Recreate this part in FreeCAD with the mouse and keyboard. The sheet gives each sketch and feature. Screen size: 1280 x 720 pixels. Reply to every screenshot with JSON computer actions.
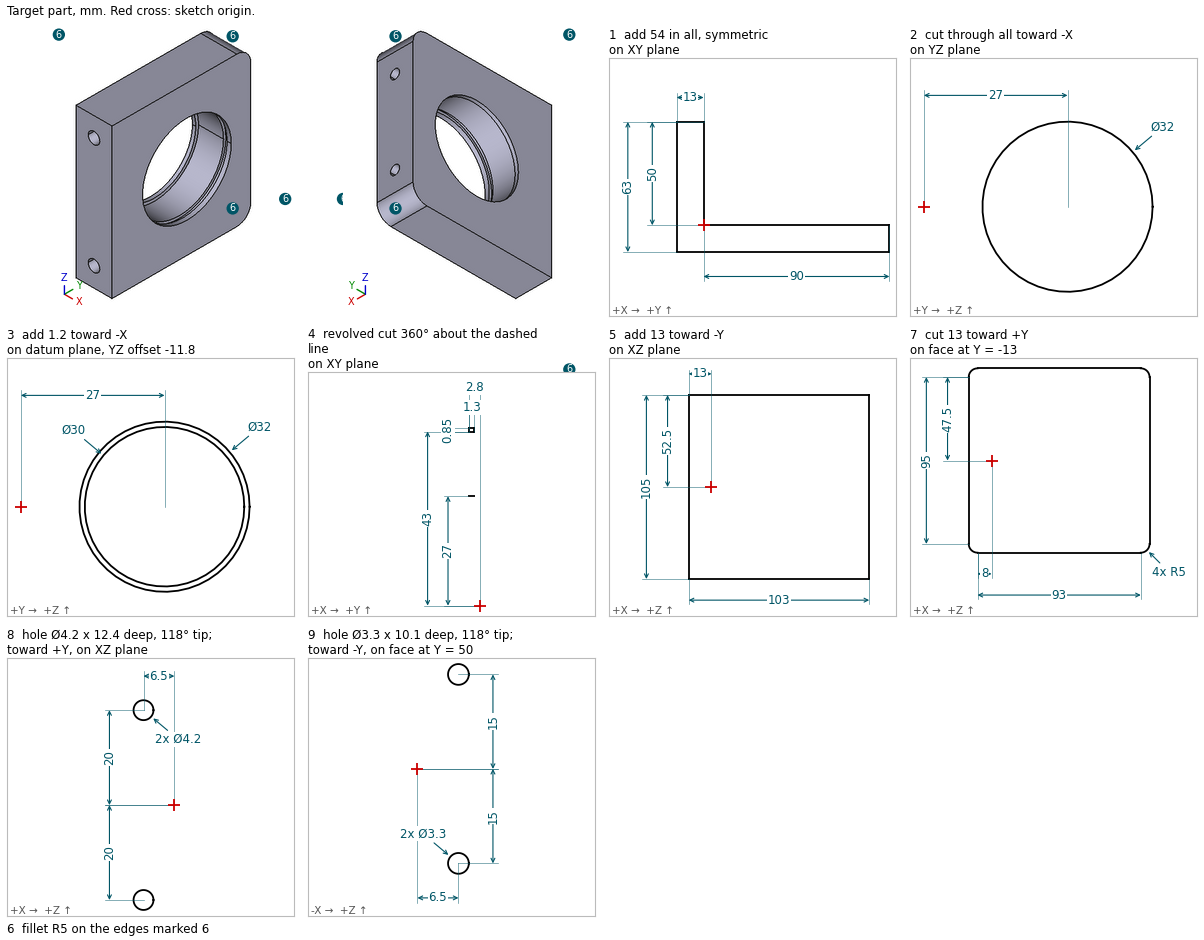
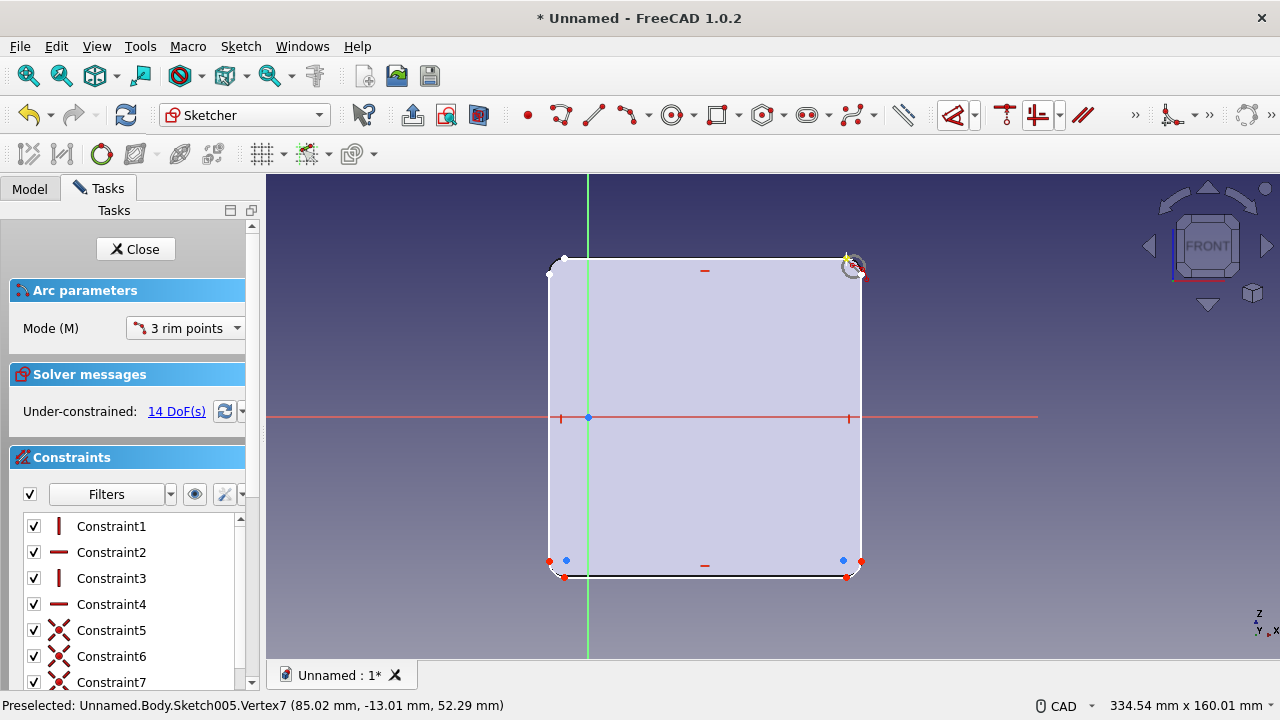
{"action": "scroll", "coordinate": [857, 263], "scroll_direction": "up", "scroll_amount": 7}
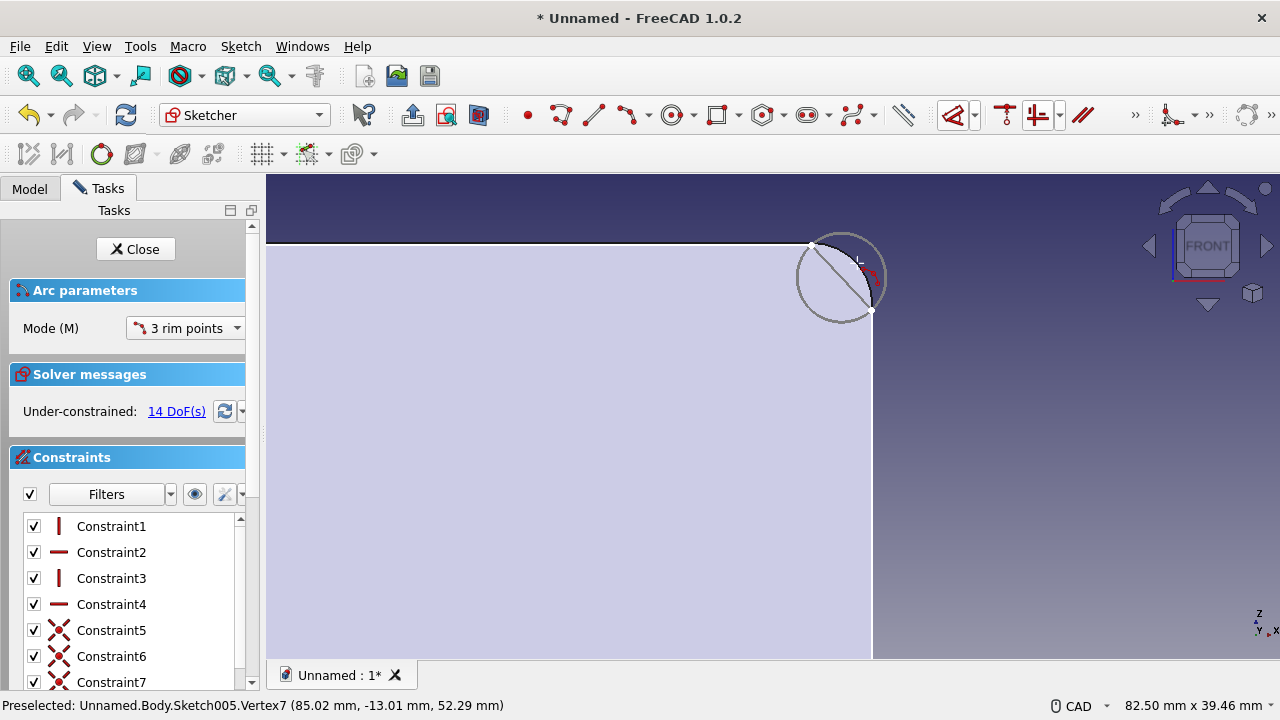
{"action": "left_click", "coordinate": [854, 261]}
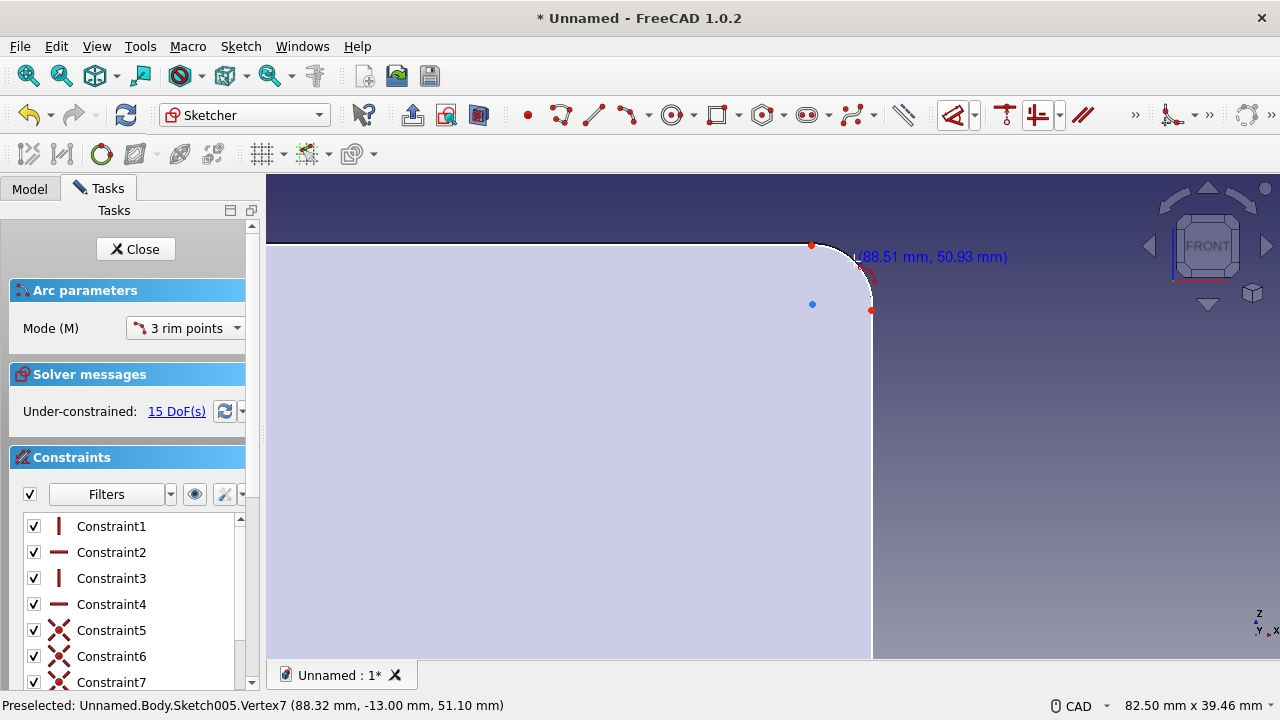
{"action": "scroll", "coordinate": [857, 262], "scroll_direction": "down", "scroll_amount": 7}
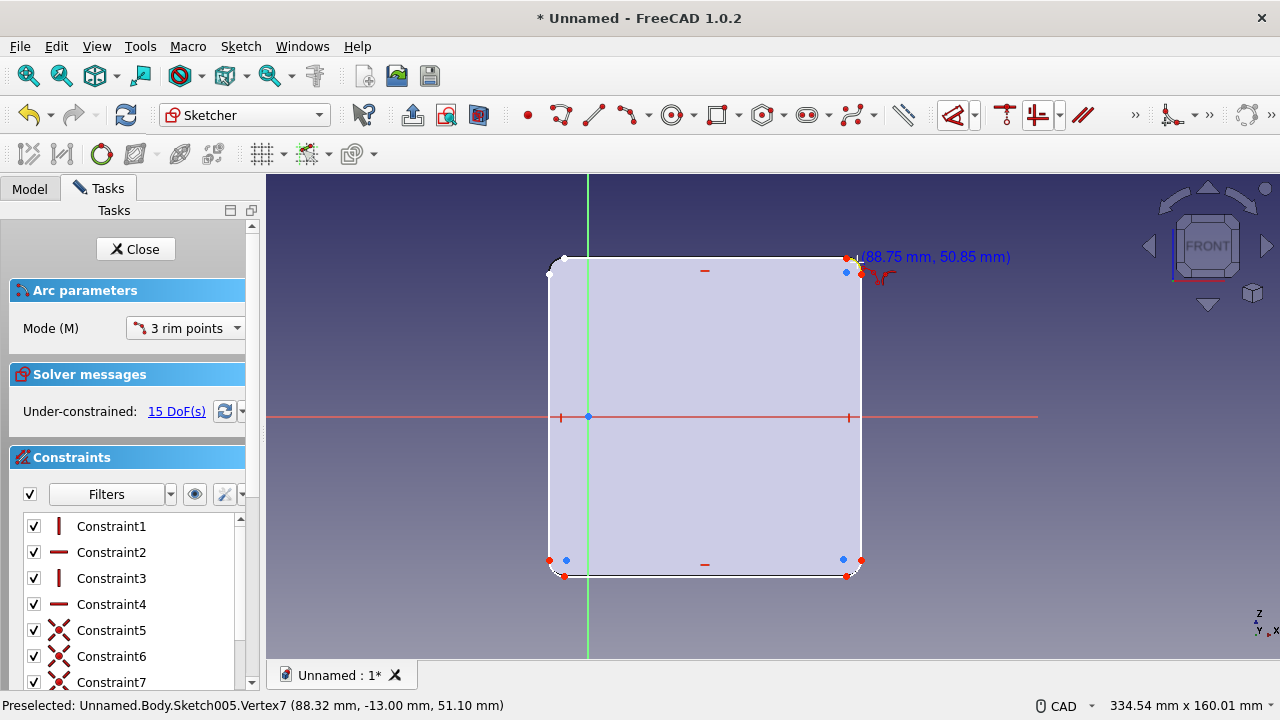
{"action": "left_click", "coordinate": [564, 258]}
{"action": "left_click", "coordinate": [549, 274]}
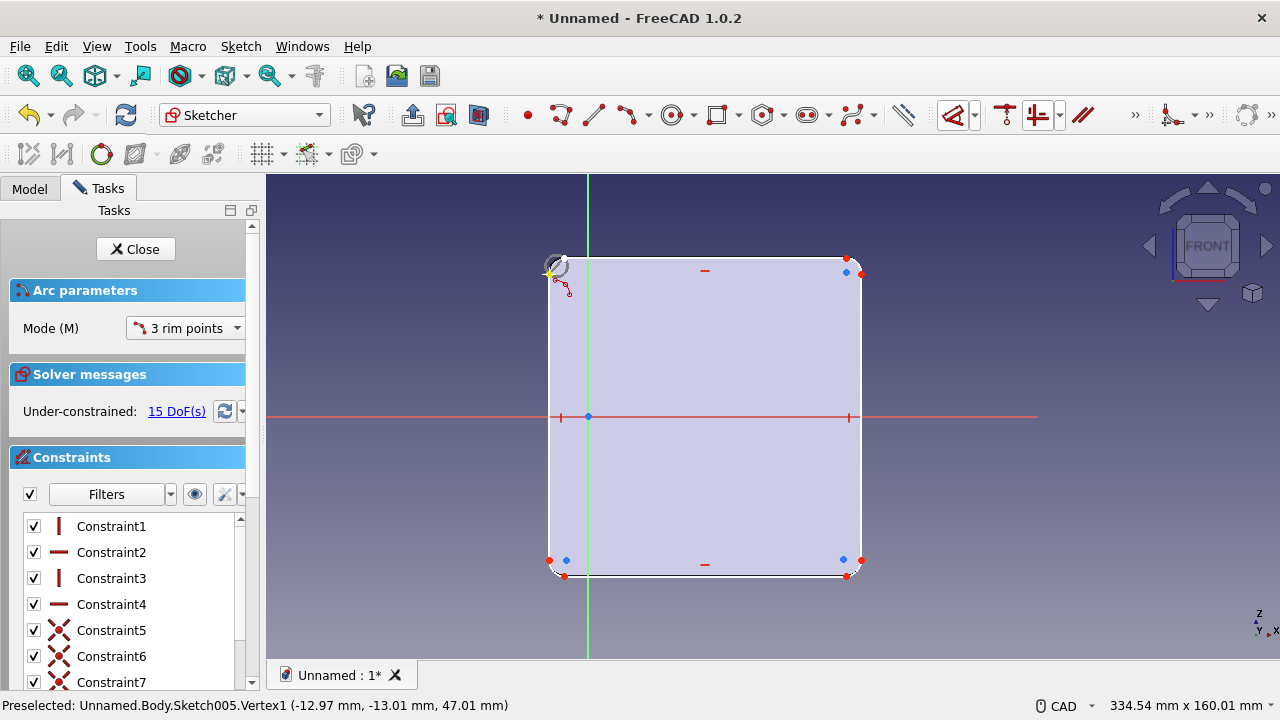
{"action": "scroll", "coordinate": [553, 262], "scroll_direction": "up", "scroll_amount": 7}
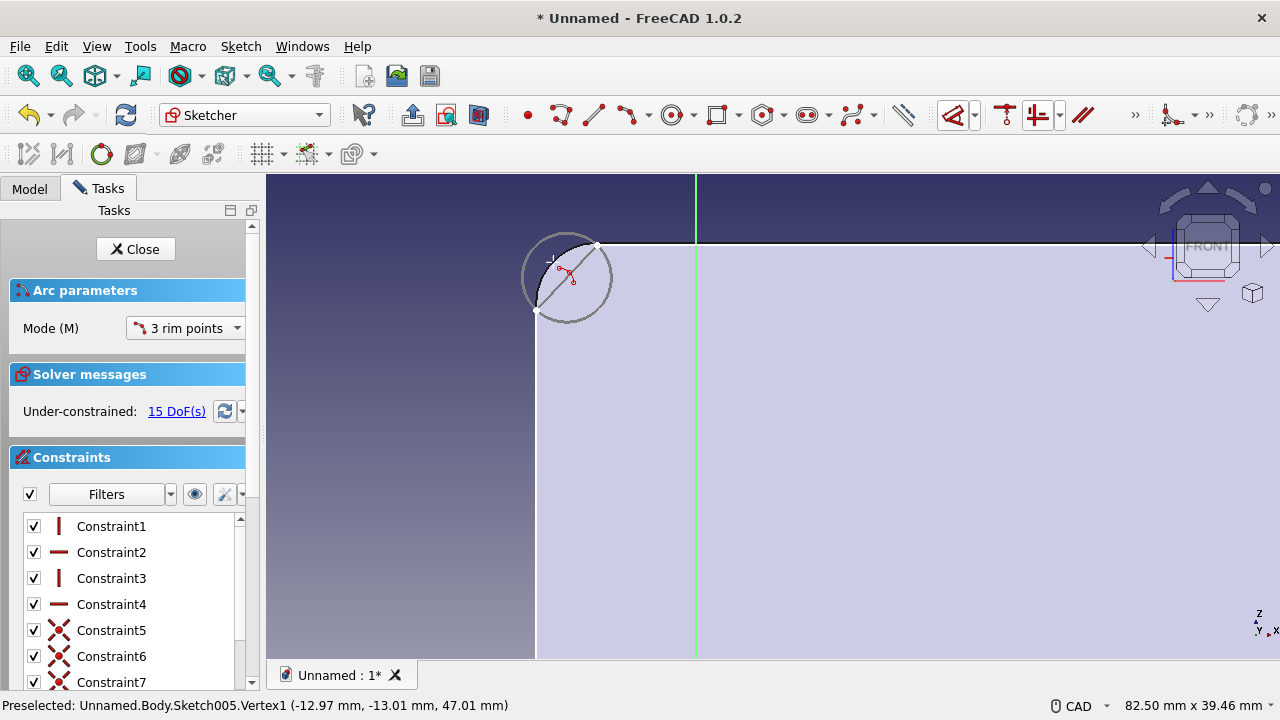
{"action": "left_click", "coordinate": [554, 261]}
{"action": "key", "text": "Escape"}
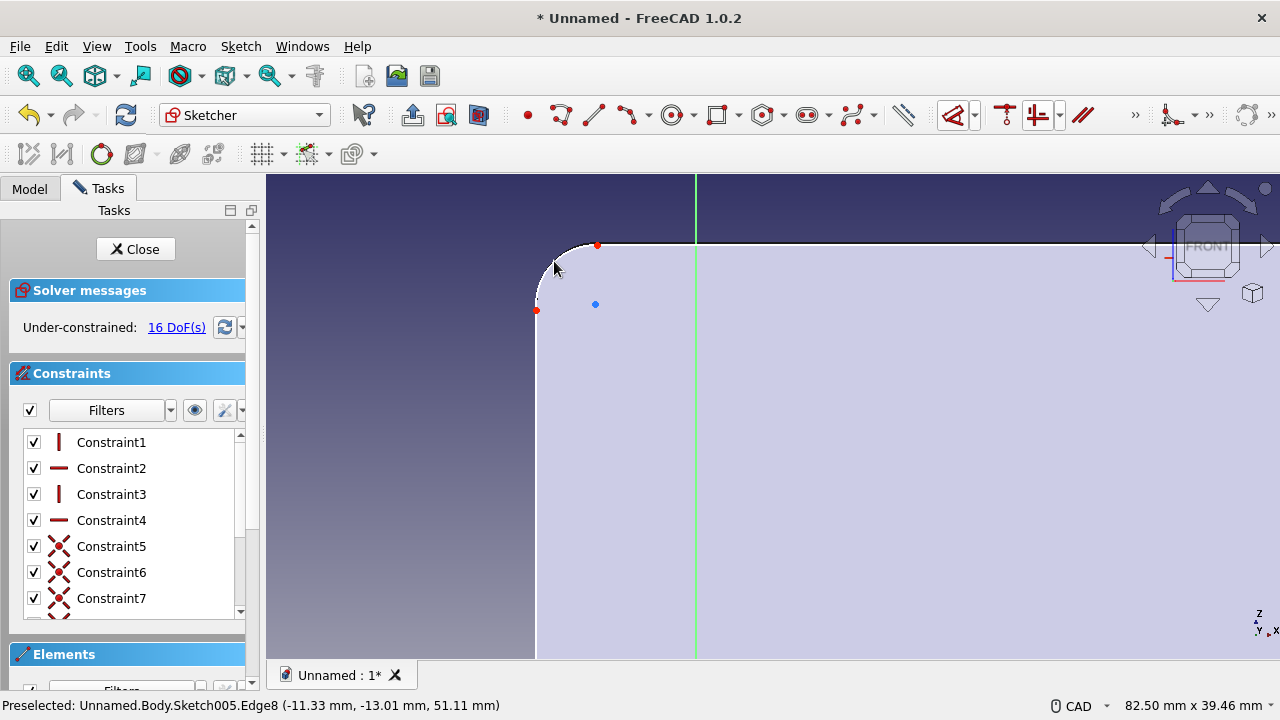
{"action": "scroll", "coordinate": [552, 262], "scroll_direction": "down", "scroll_amount": 7}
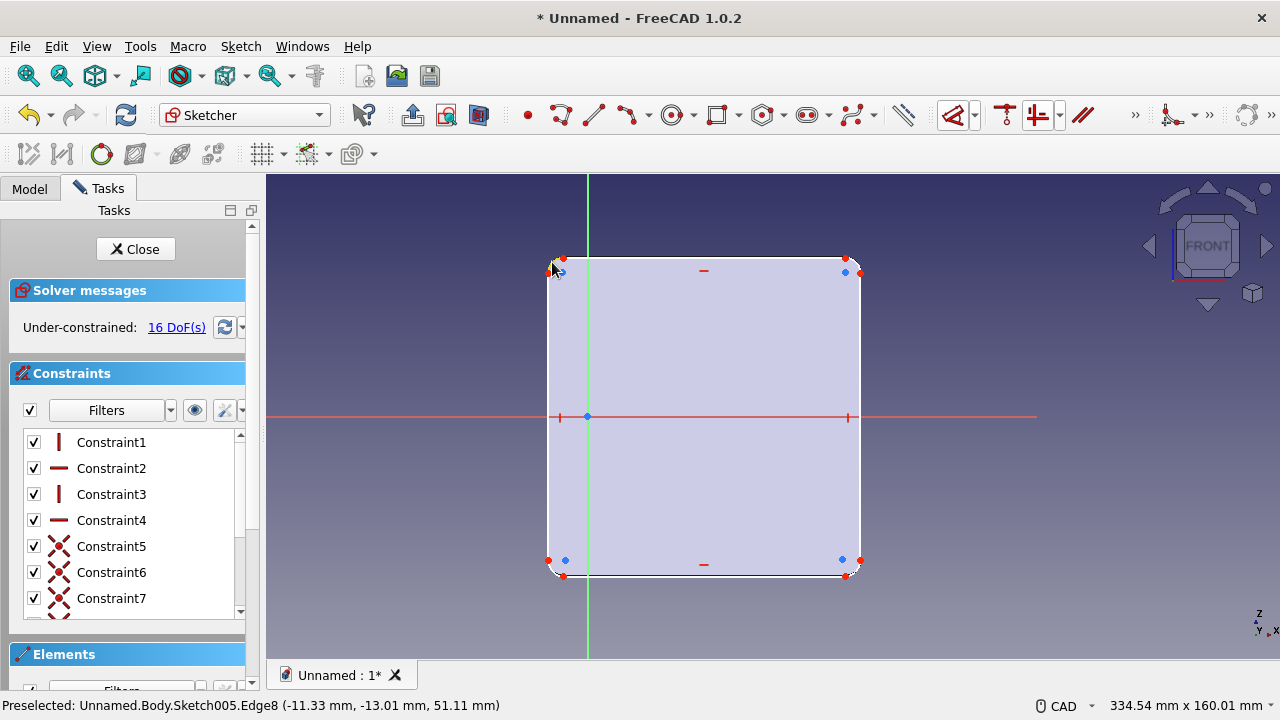
{"action": "left_click", "coordinate": [548, 331]}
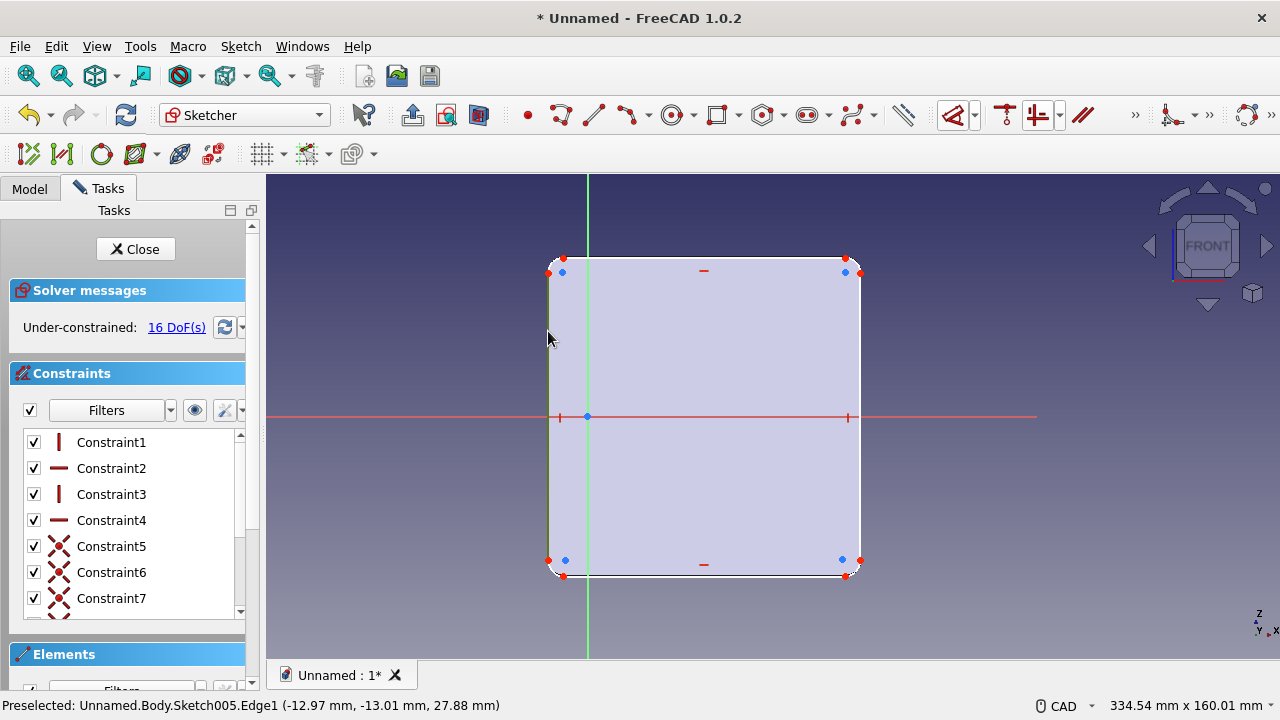
{"action": "left_click", "coordinate": [553, 572]}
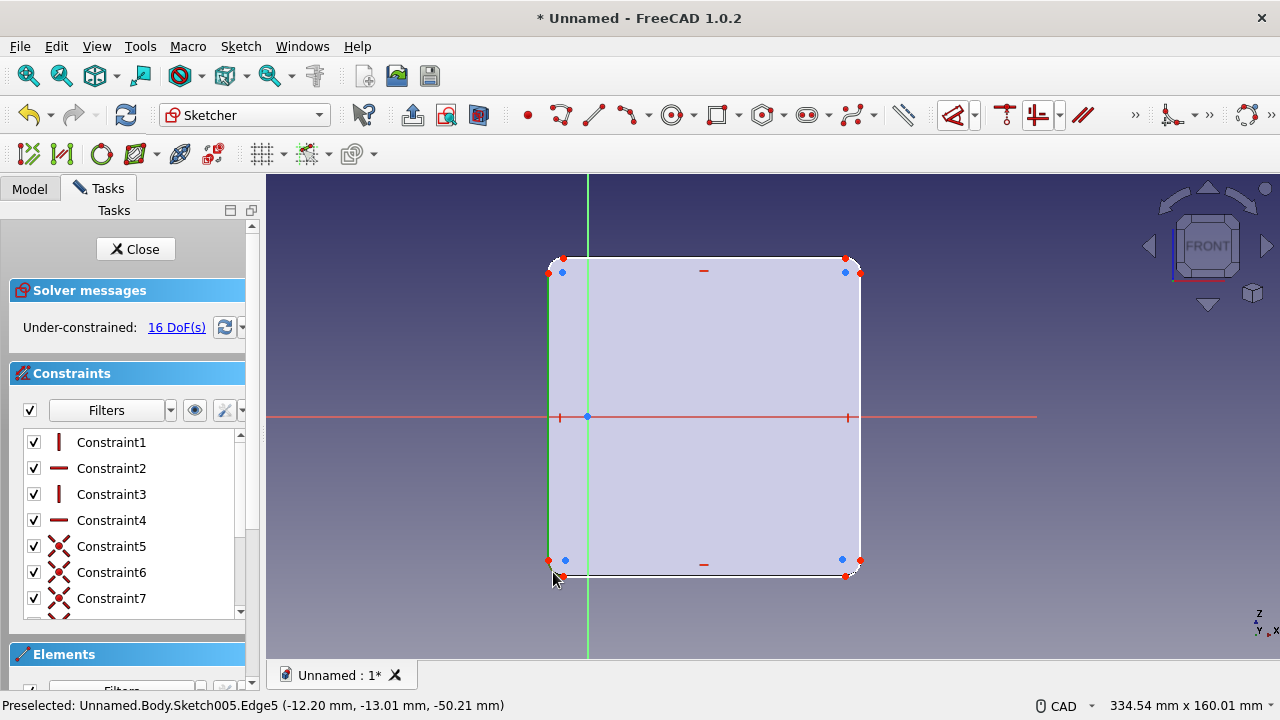
{"action": "key", "text": "t"}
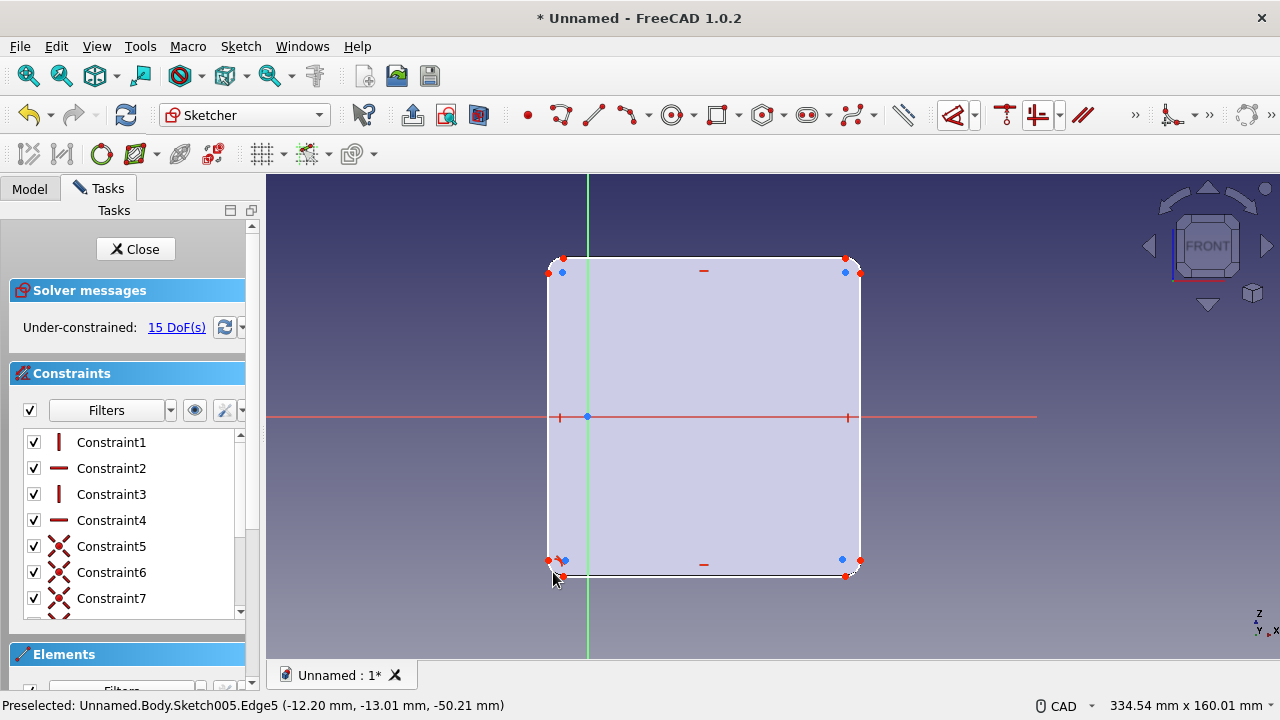
{"action": "left_click", "coordinate": [548, 360]}